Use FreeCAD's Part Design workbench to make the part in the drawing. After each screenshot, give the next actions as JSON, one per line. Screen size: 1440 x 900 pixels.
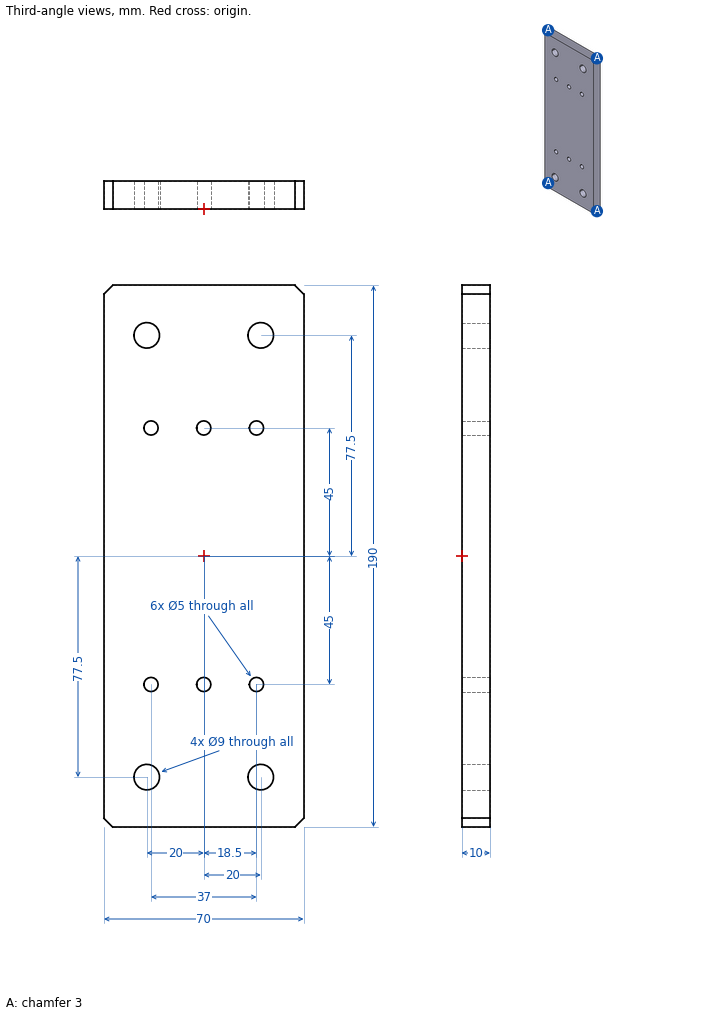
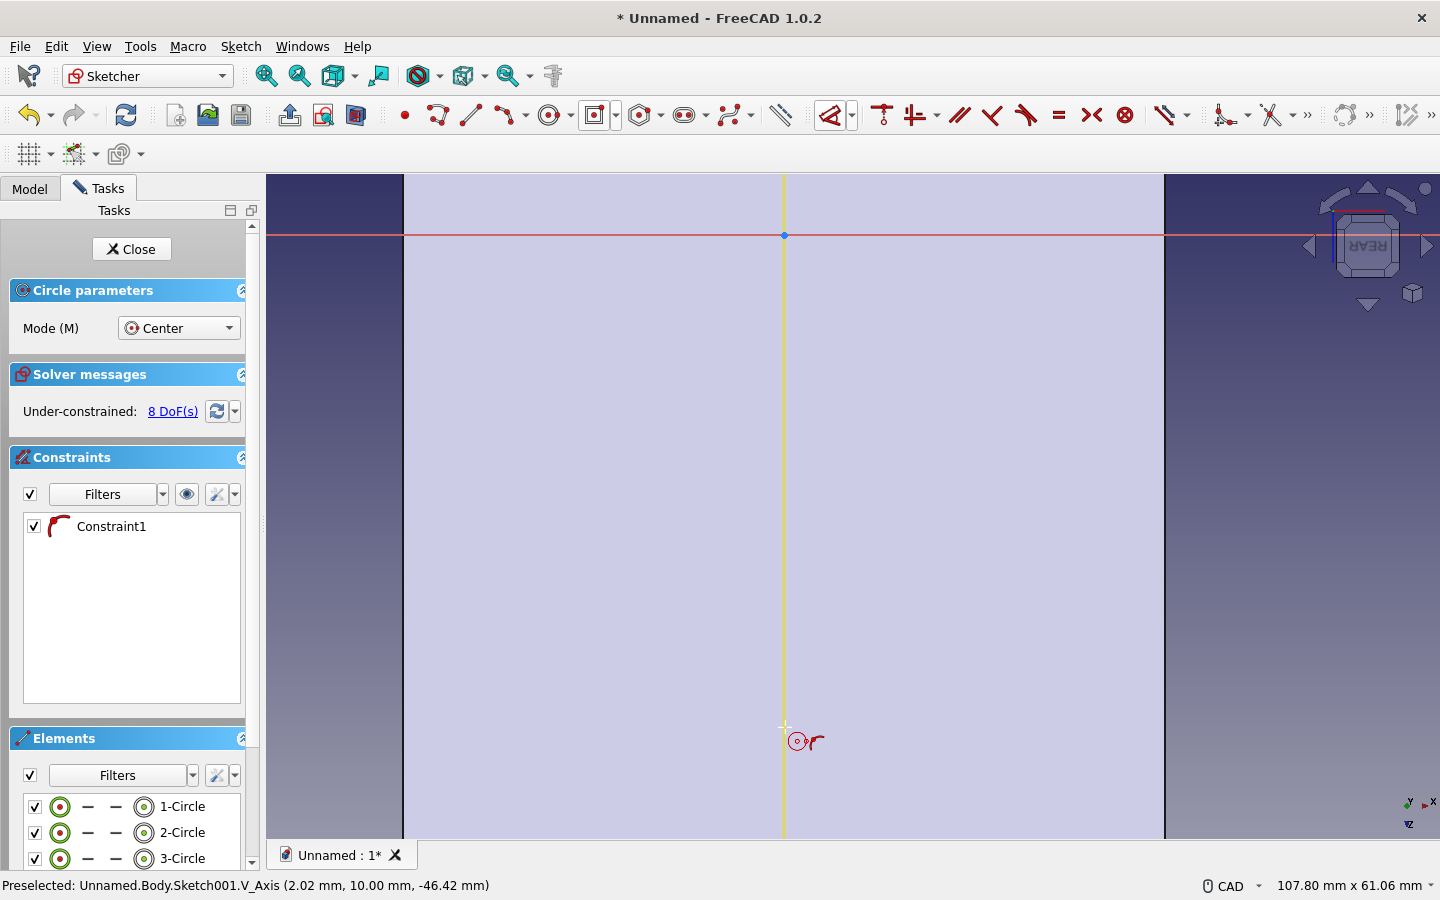
{"action": "left_click", "coordinate": [784, 725]}
{"action": "left_click", "coordinate": [803, 706]}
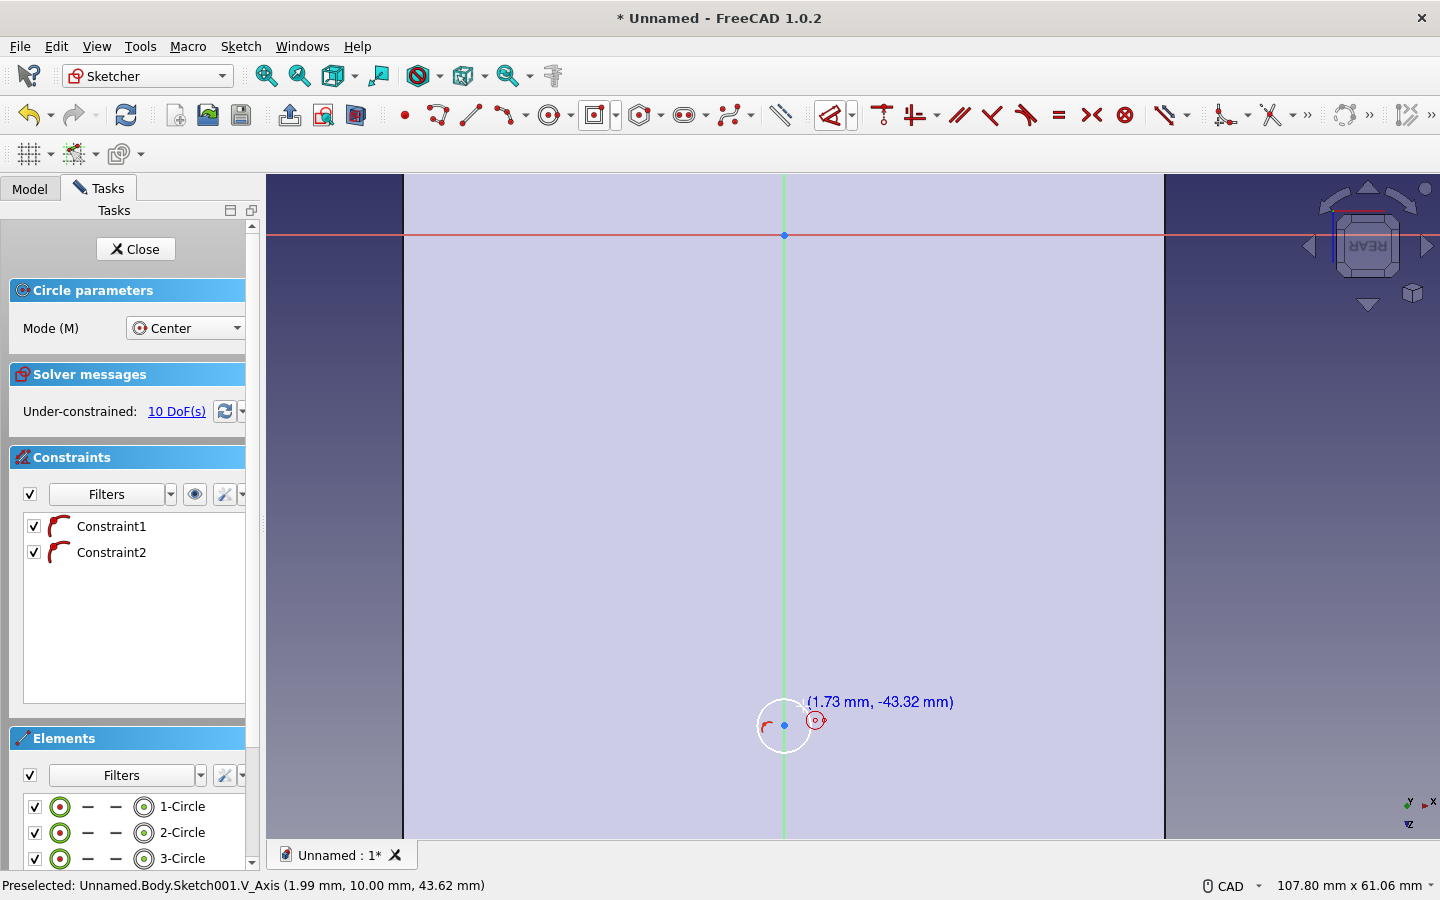
{"action": "left_click", "coordinate": [583, 725]}
{"action": "left_click", "coordinate": [602, 706]}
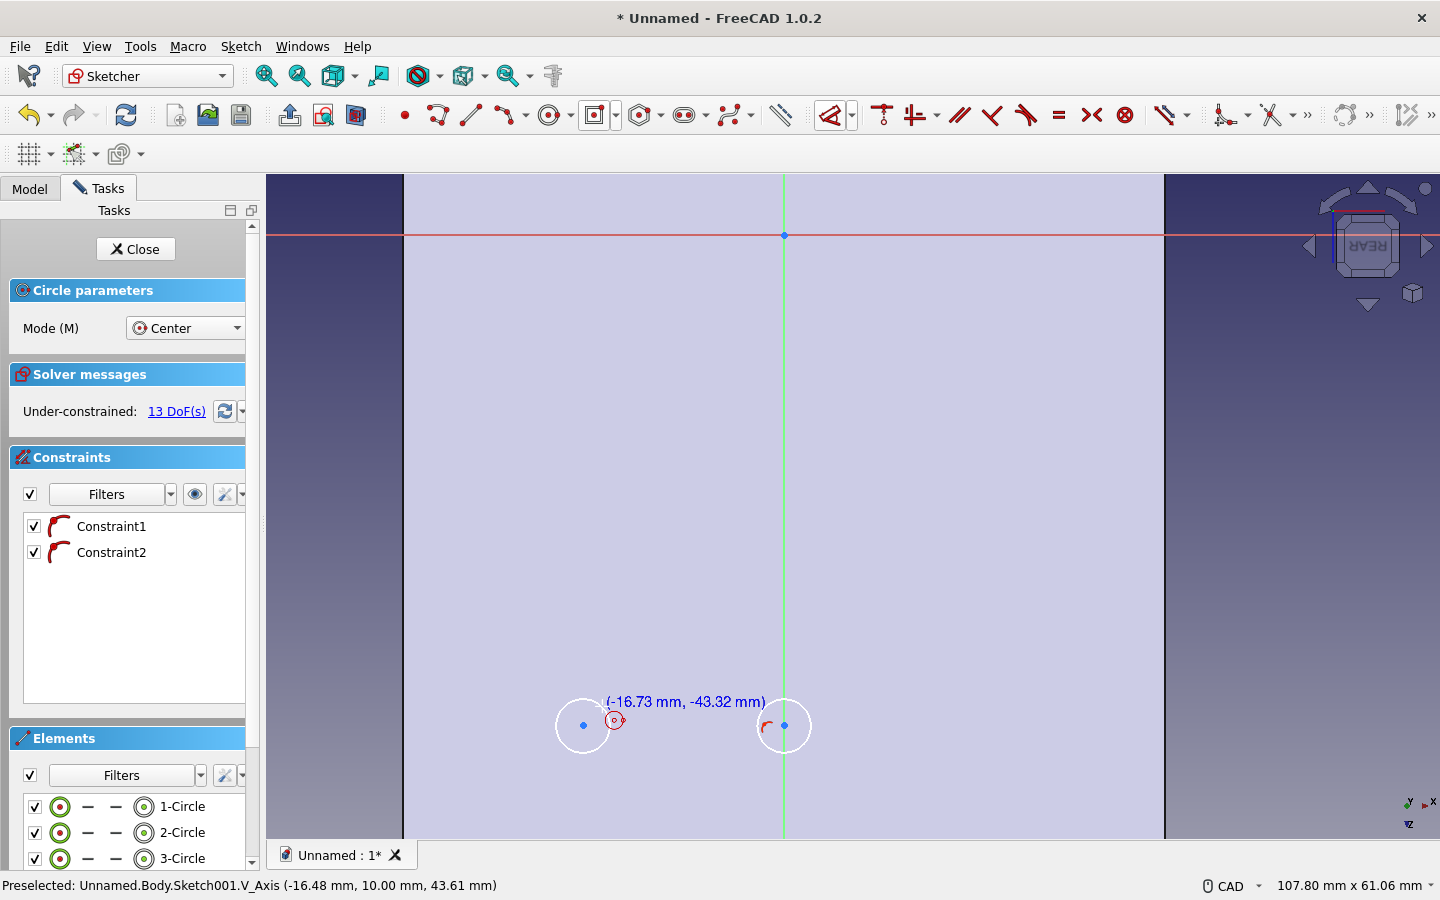
{"action": "left_click", "coordinate": [986, 725]}
{"action": "left_click", "coordinate": [1005, 706]}
{"action": "key", "text": "Escape"}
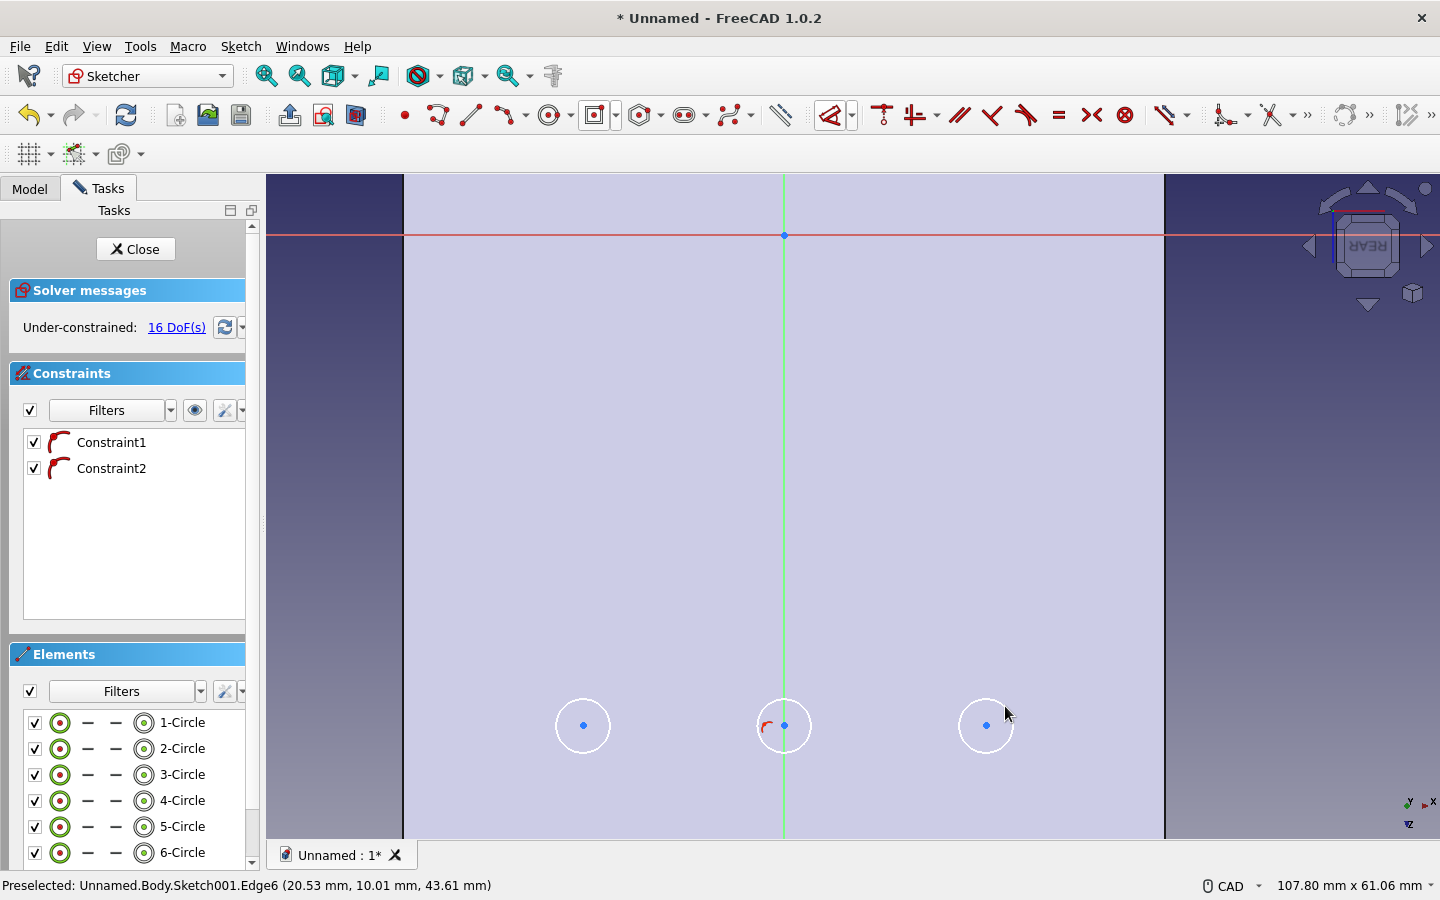
{"action": "scroll", "coordinate": [785, 728], "scroll_direction": "down", "scroll_amount": 4}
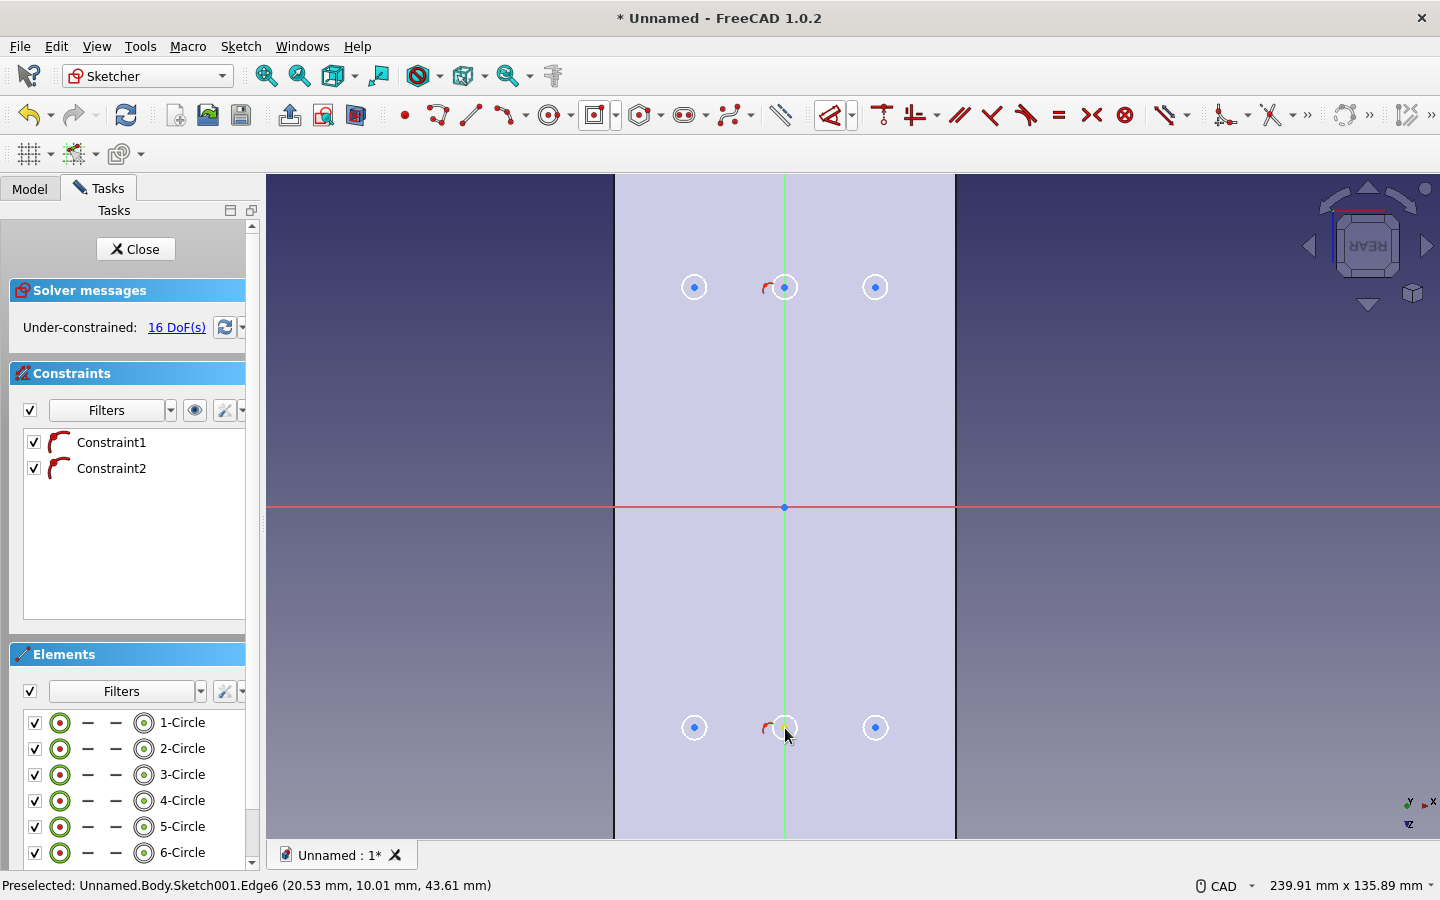
{"action": "left_click", "coordinate": [884, 279]}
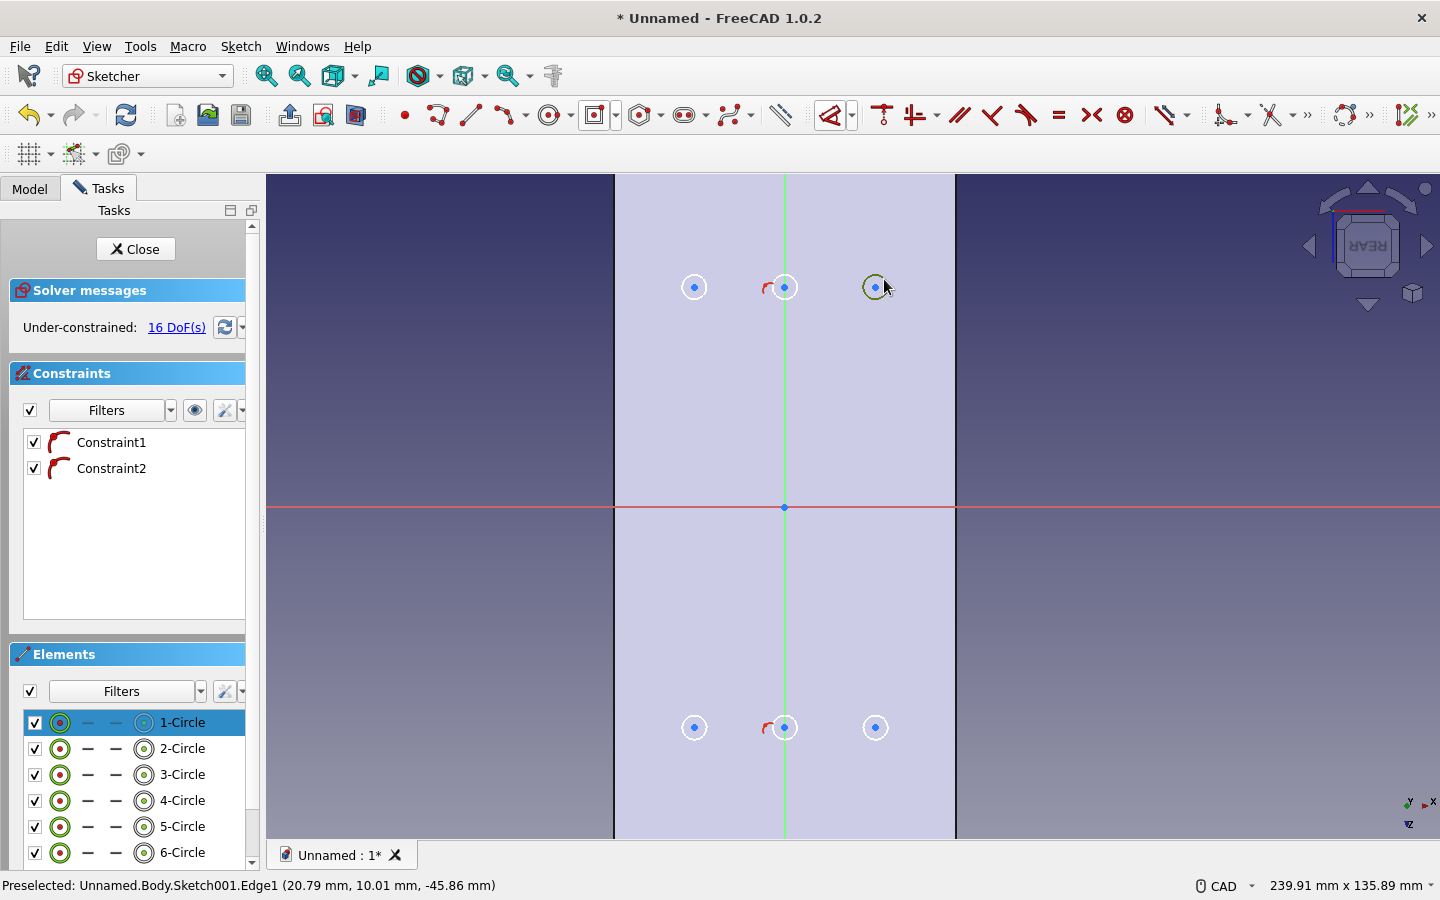
{"action": "left_click", "coordinate": [703, 279]}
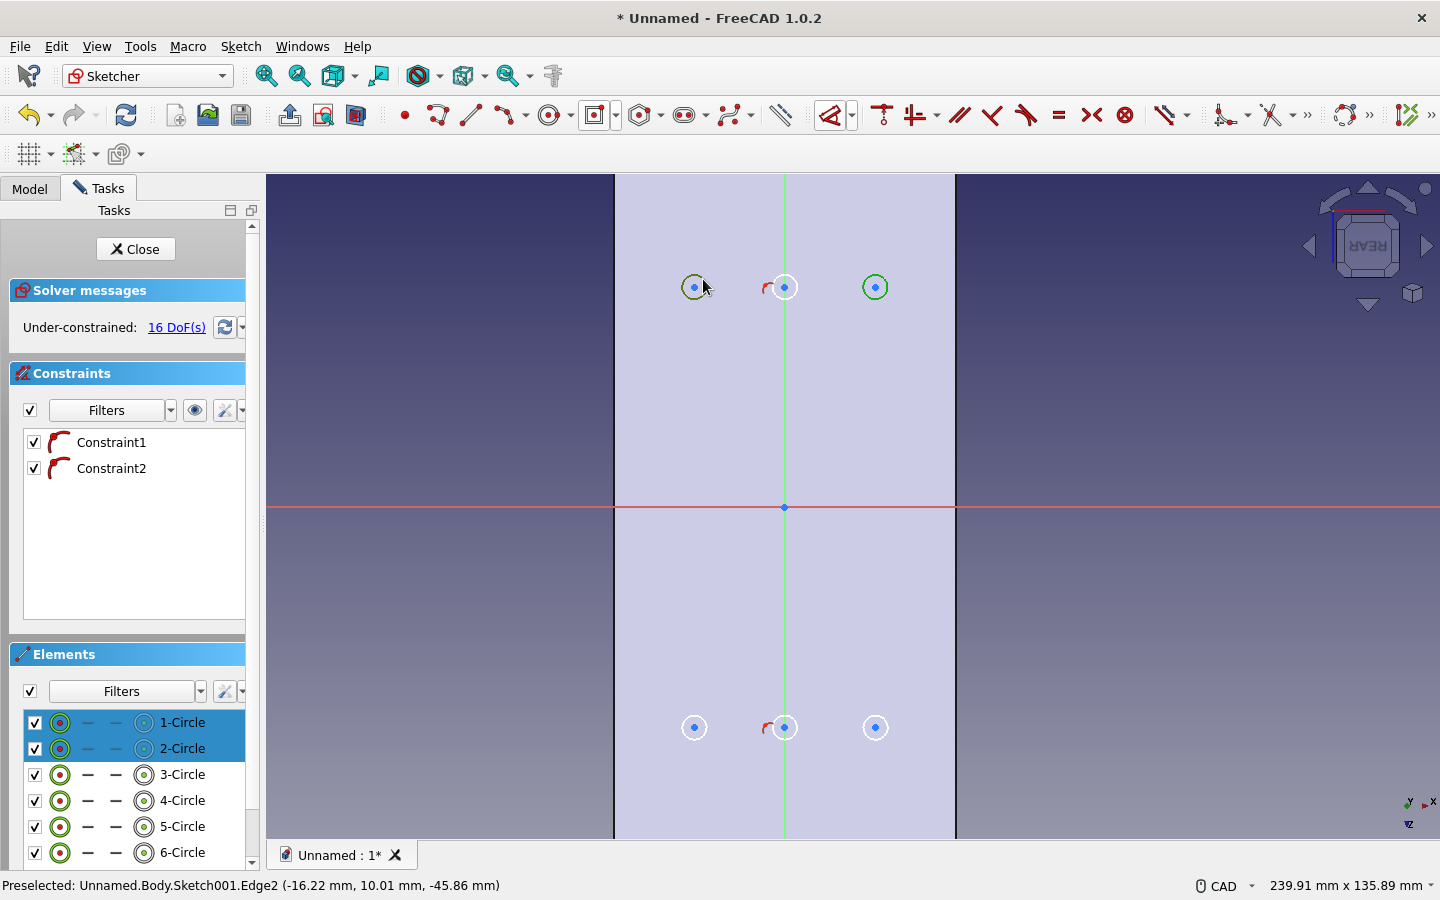
{"action": "left_click", "coordinate": [785, 275]}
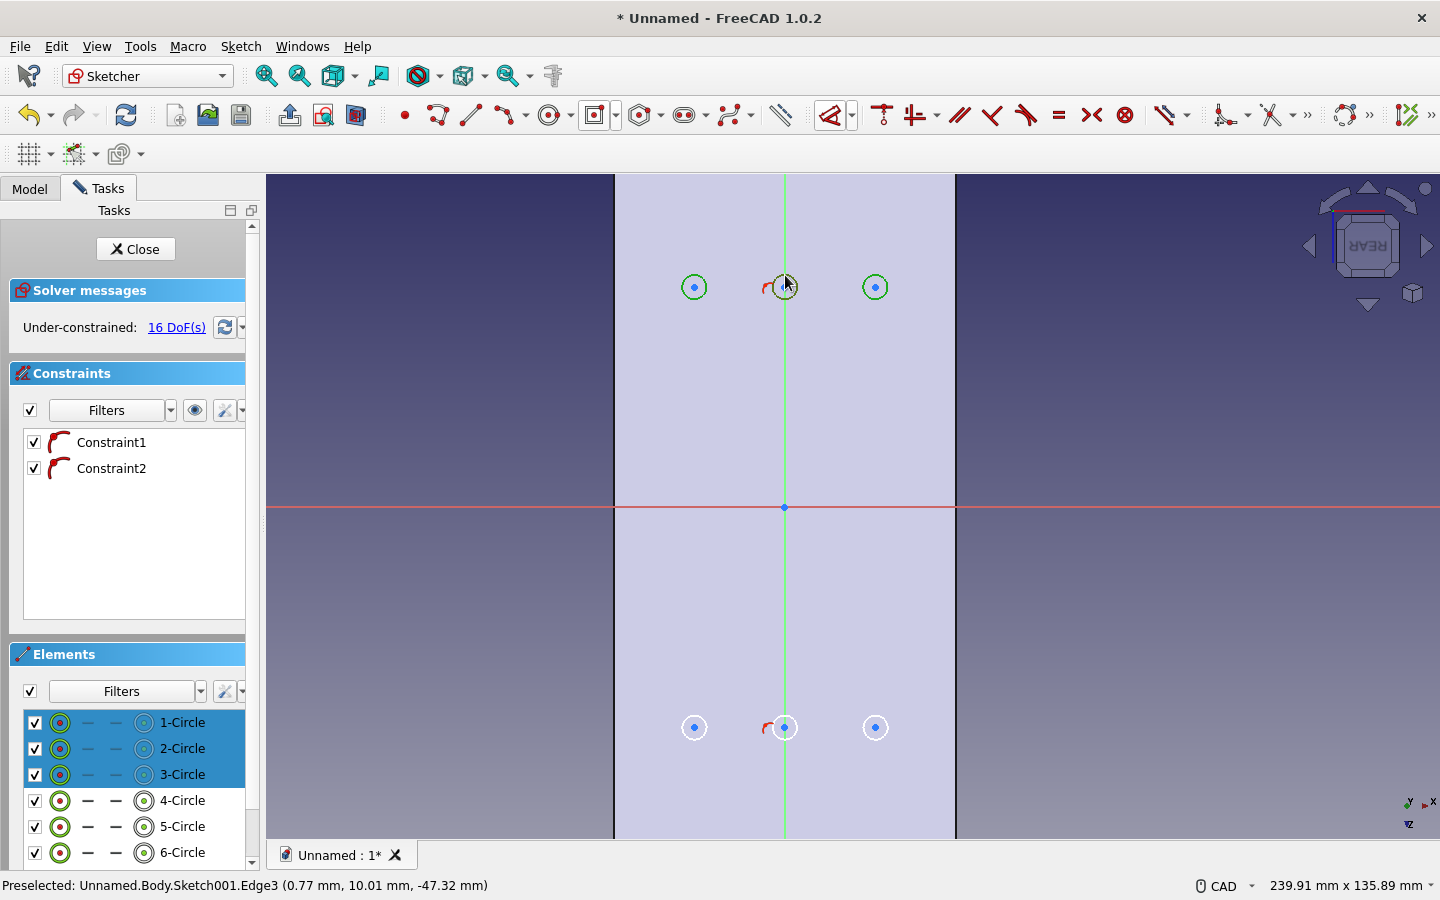
{"action": "left_click", "coordinate": [785, 716]}